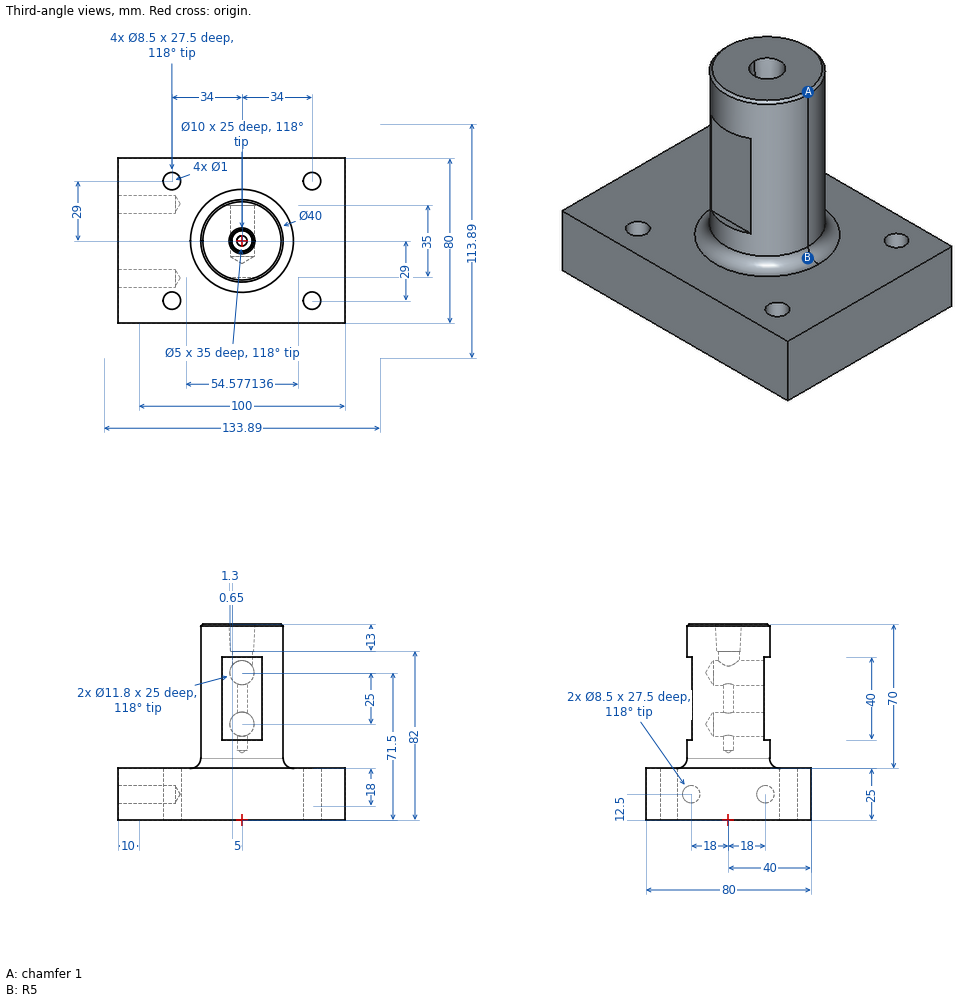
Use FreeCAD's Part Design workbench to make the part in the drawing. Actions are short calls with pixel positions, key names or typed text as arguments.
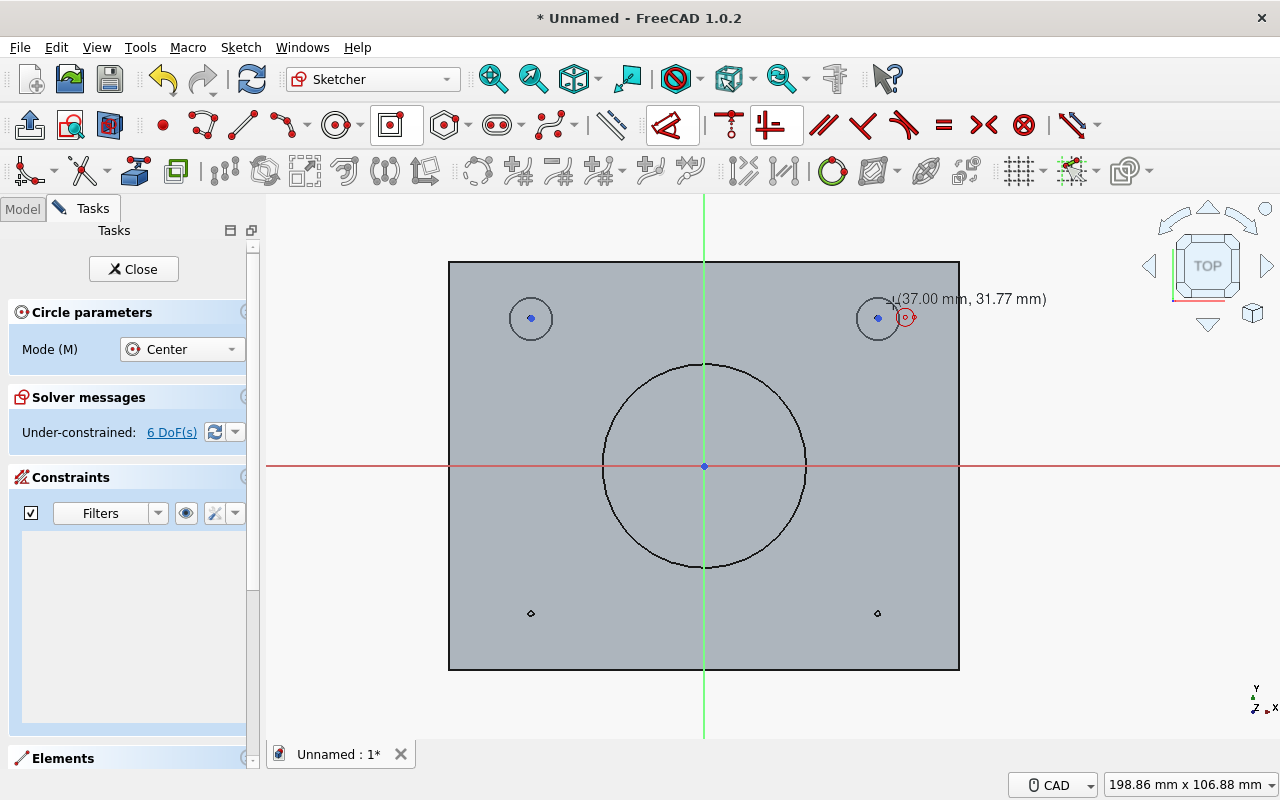
click(878, 614)
click(893, 599)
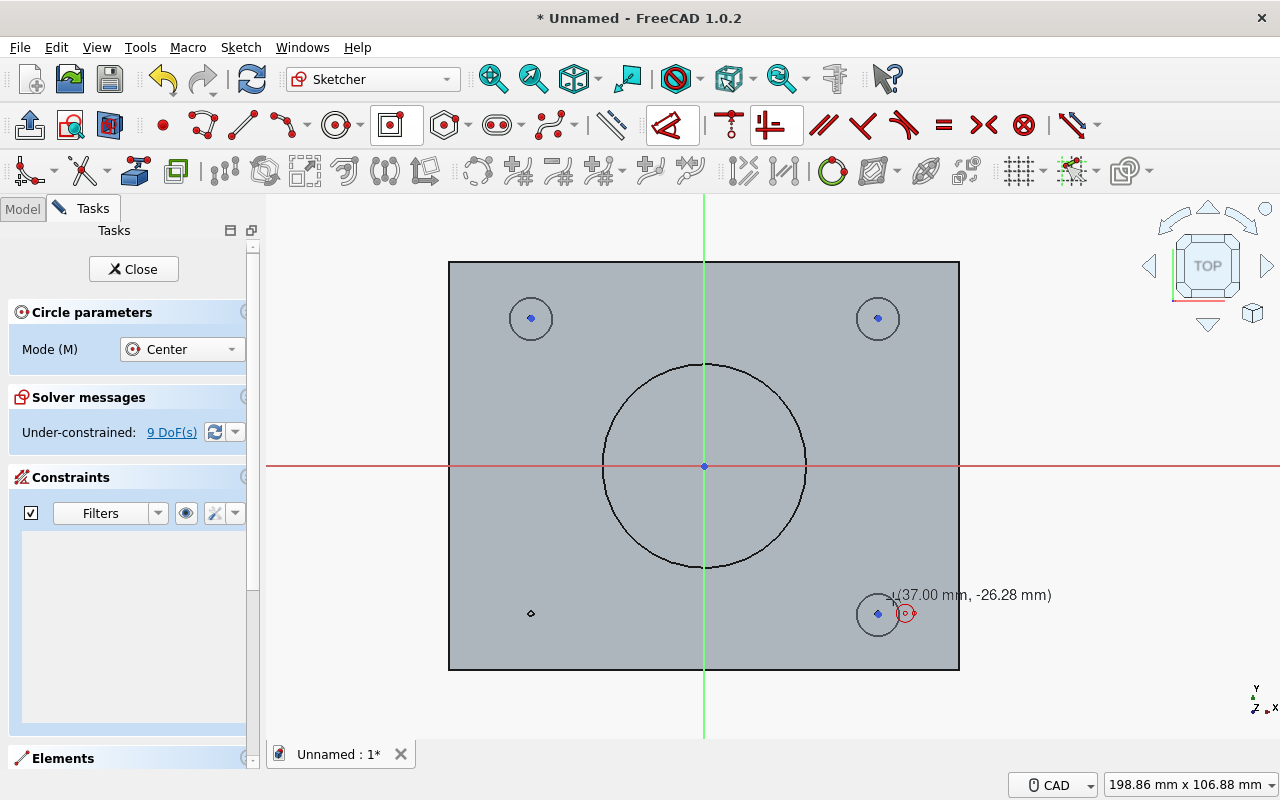
click(531, 614)
click(546, 599)
key(Escape)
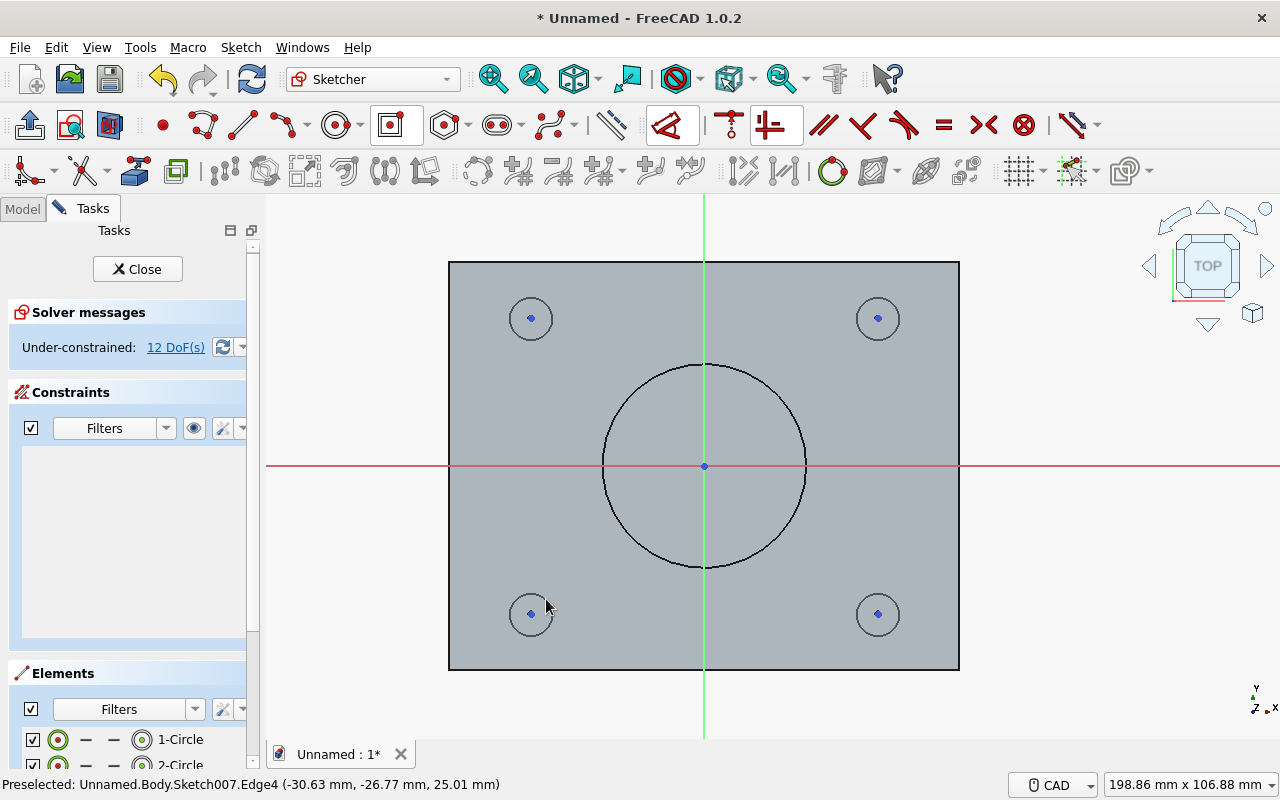
click(546, 304)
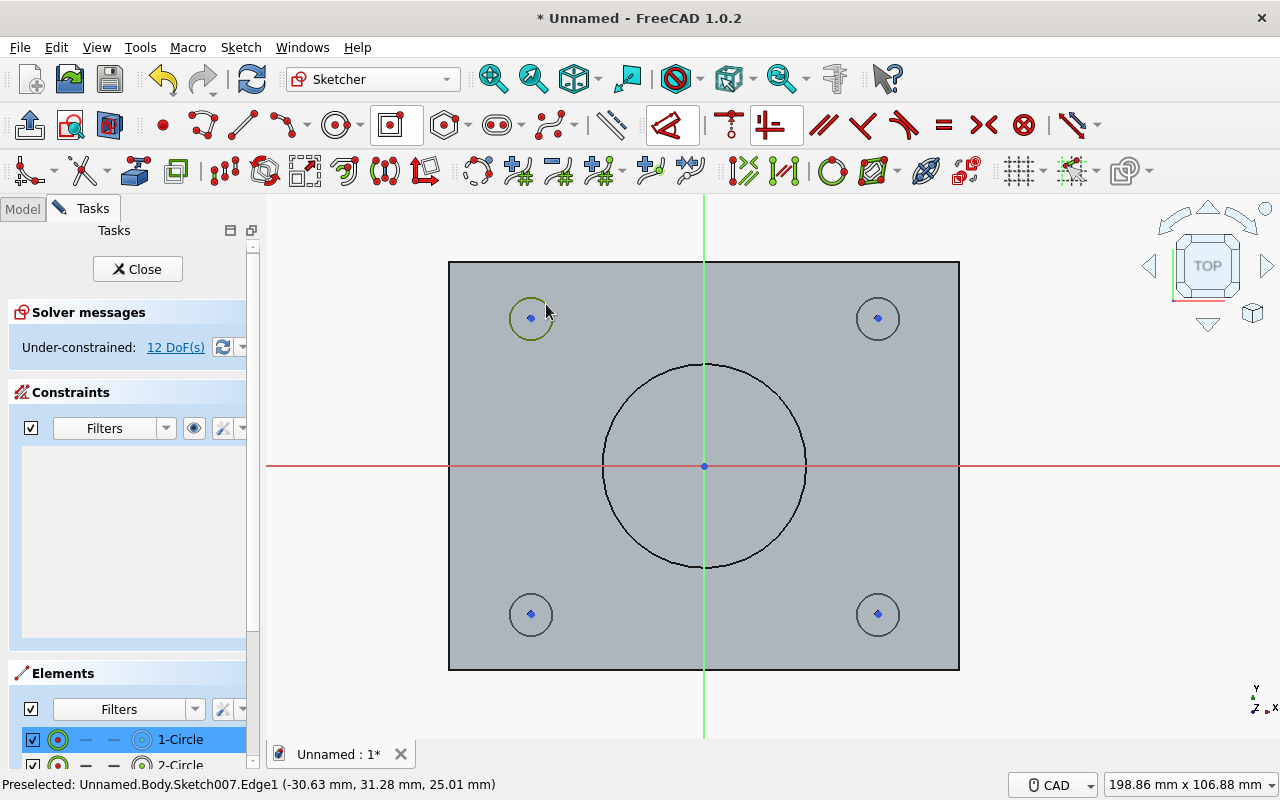
click(893, 304)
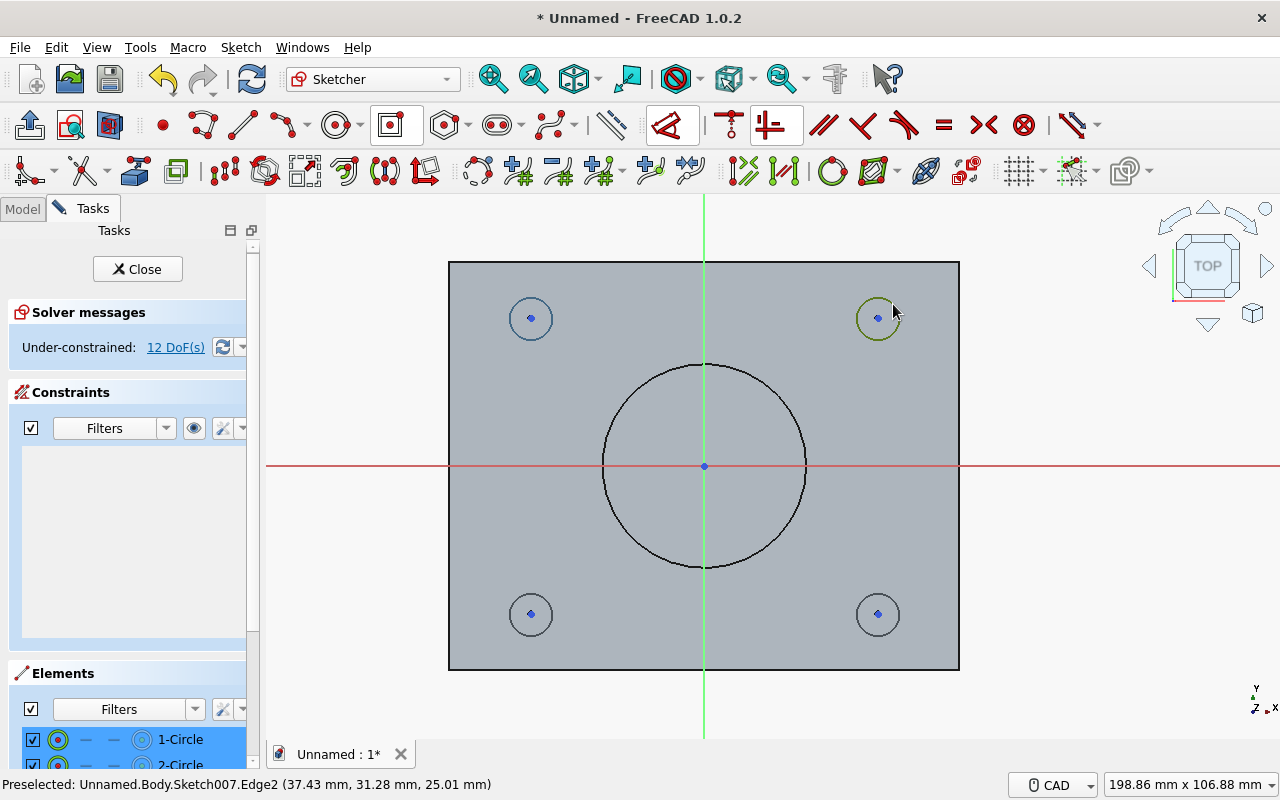
click(893, 600)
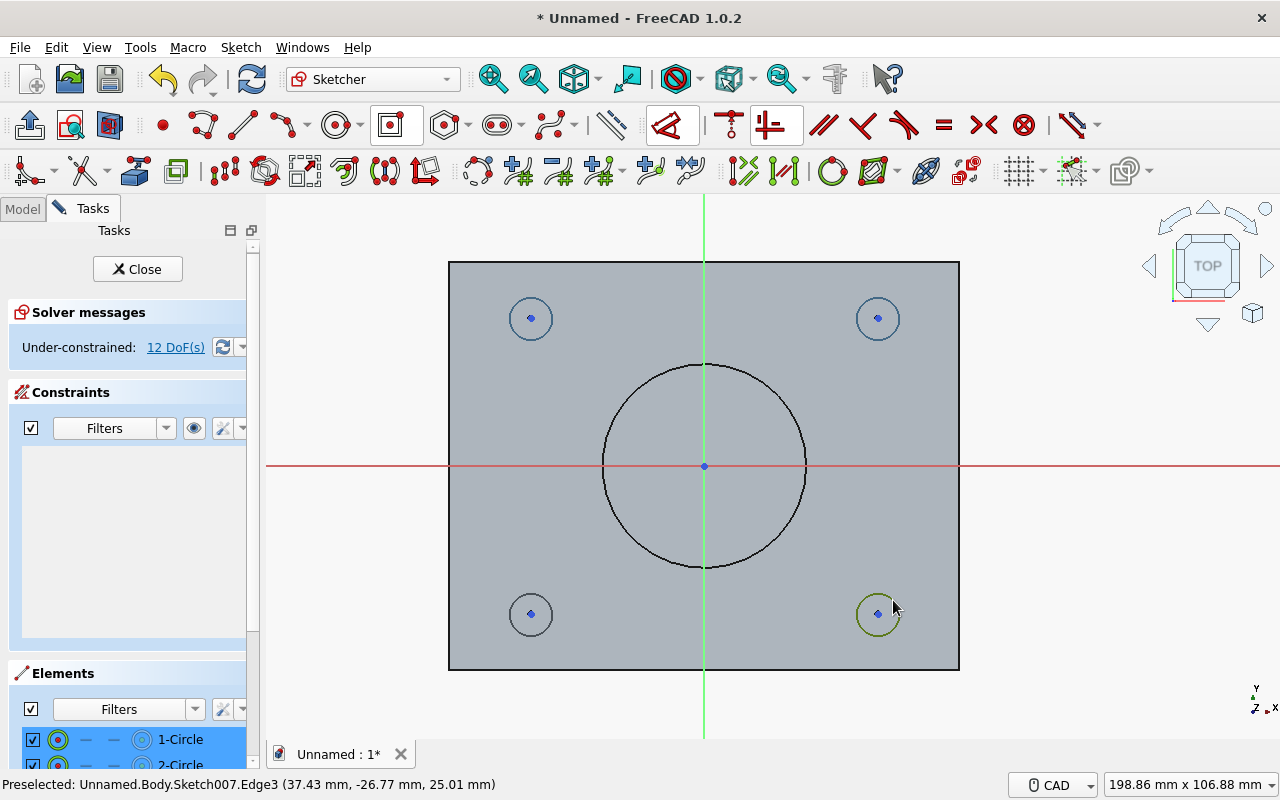
click(546, 600)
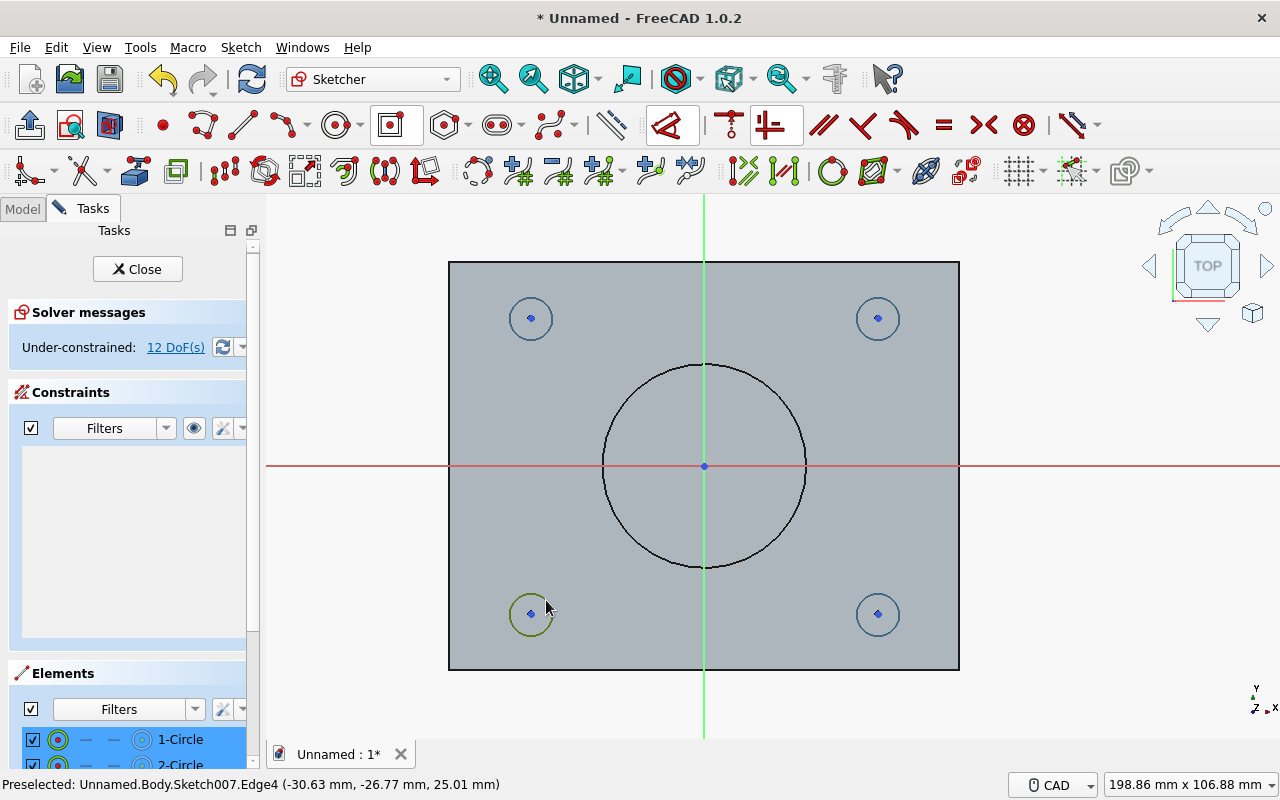
click(944, 126)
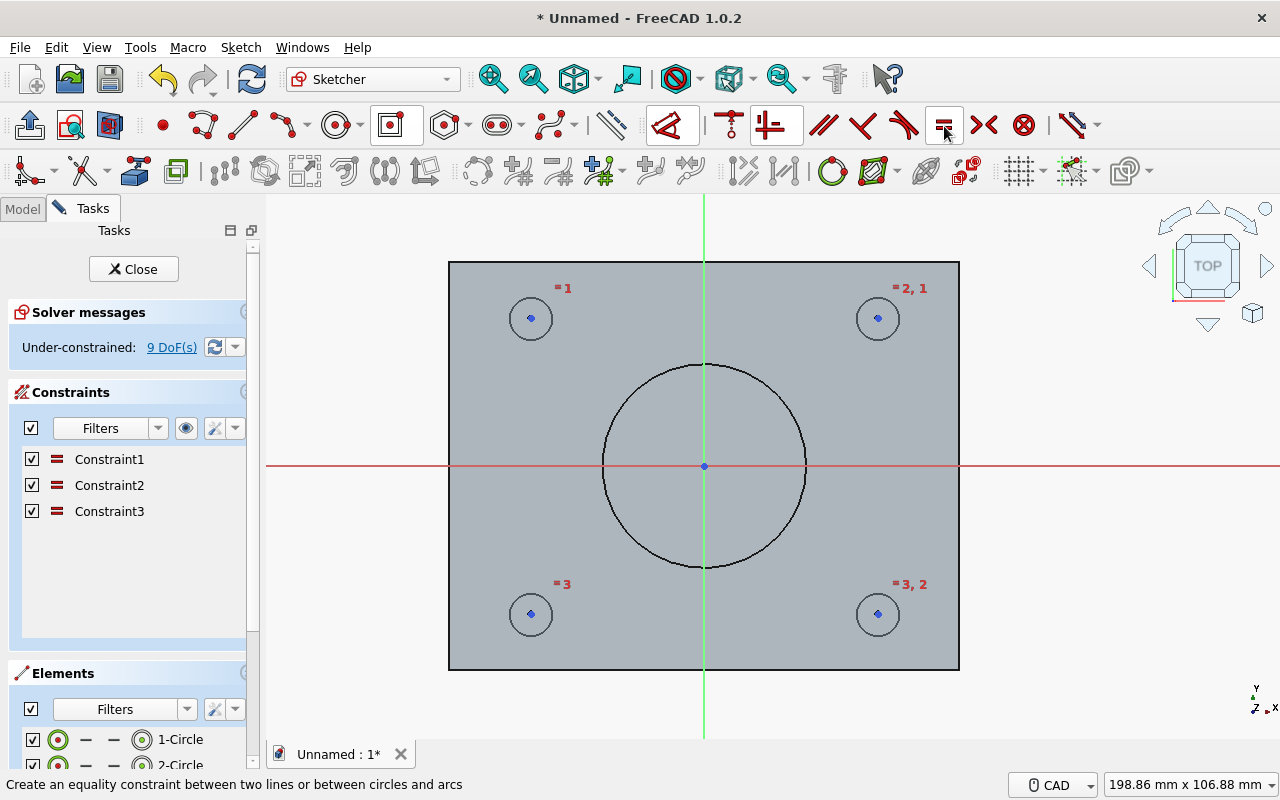
click(546, 304)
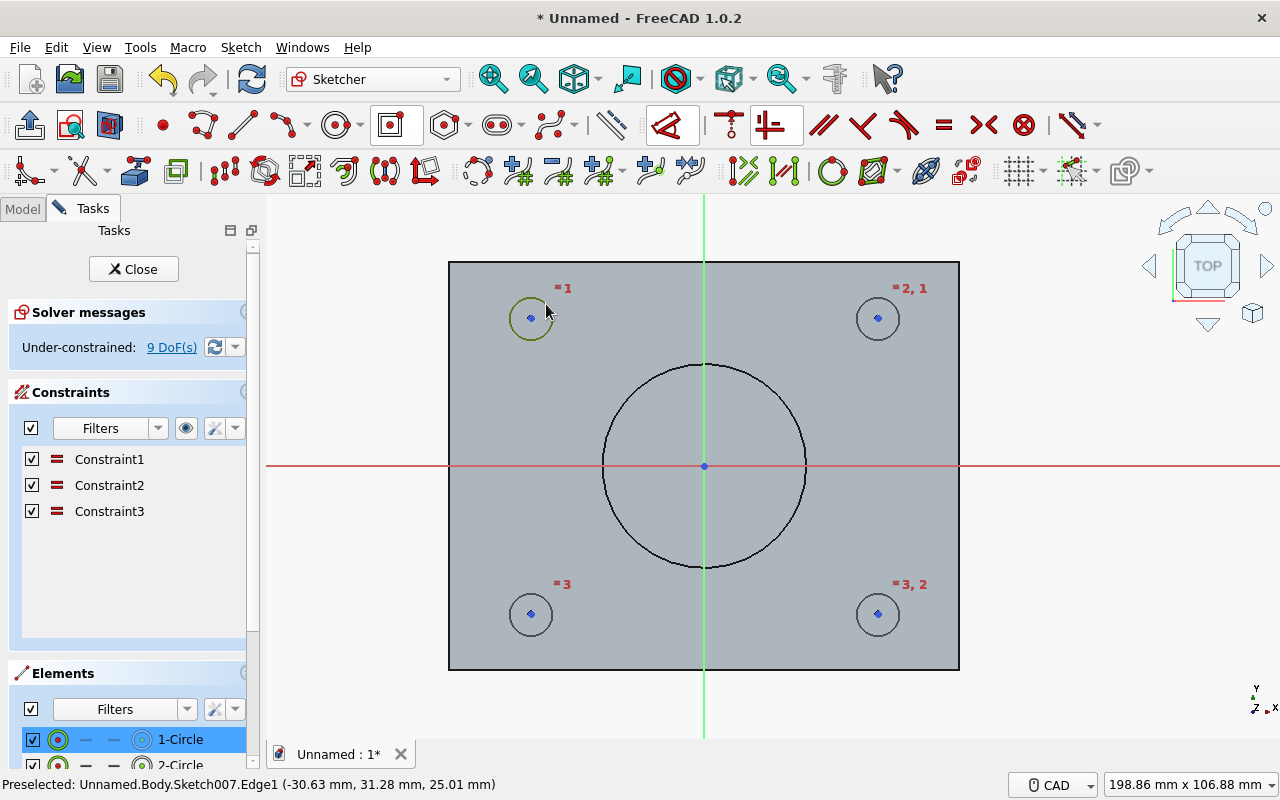
click(694, 126)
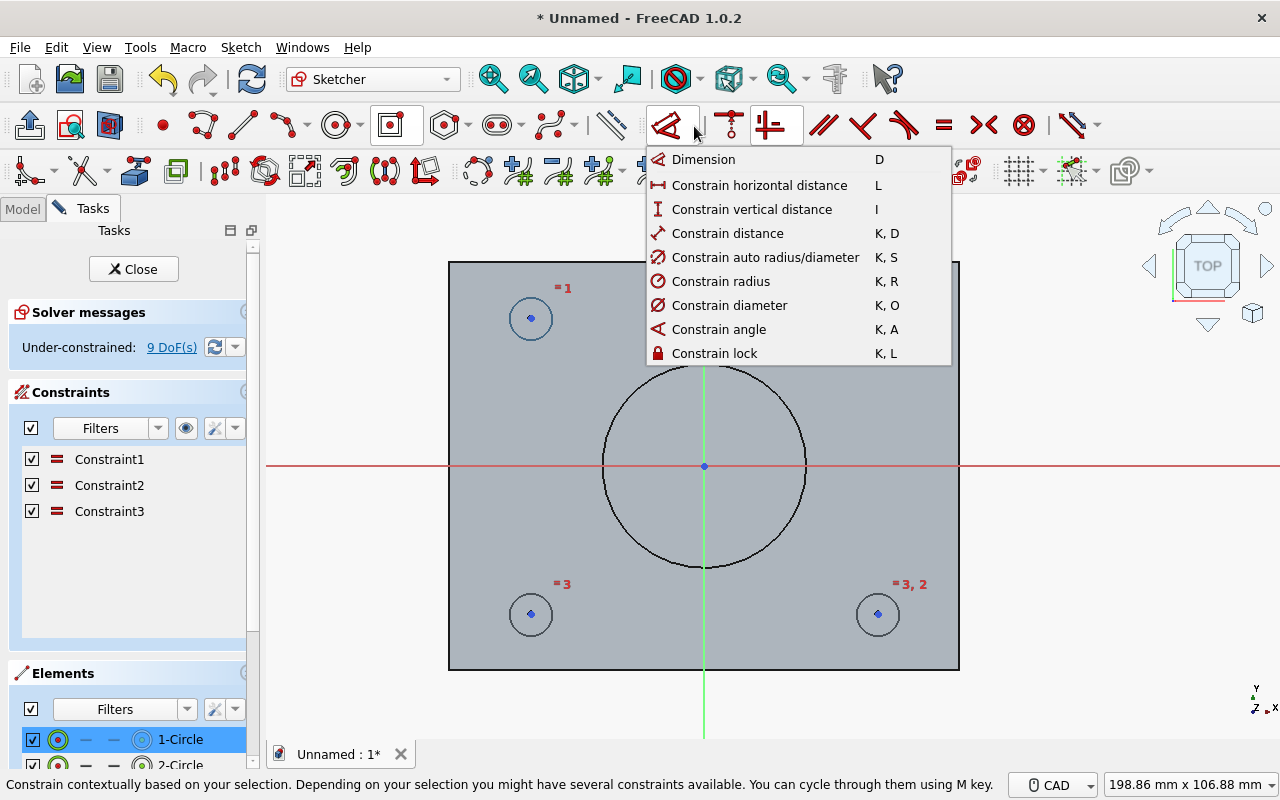
click(799, 305)